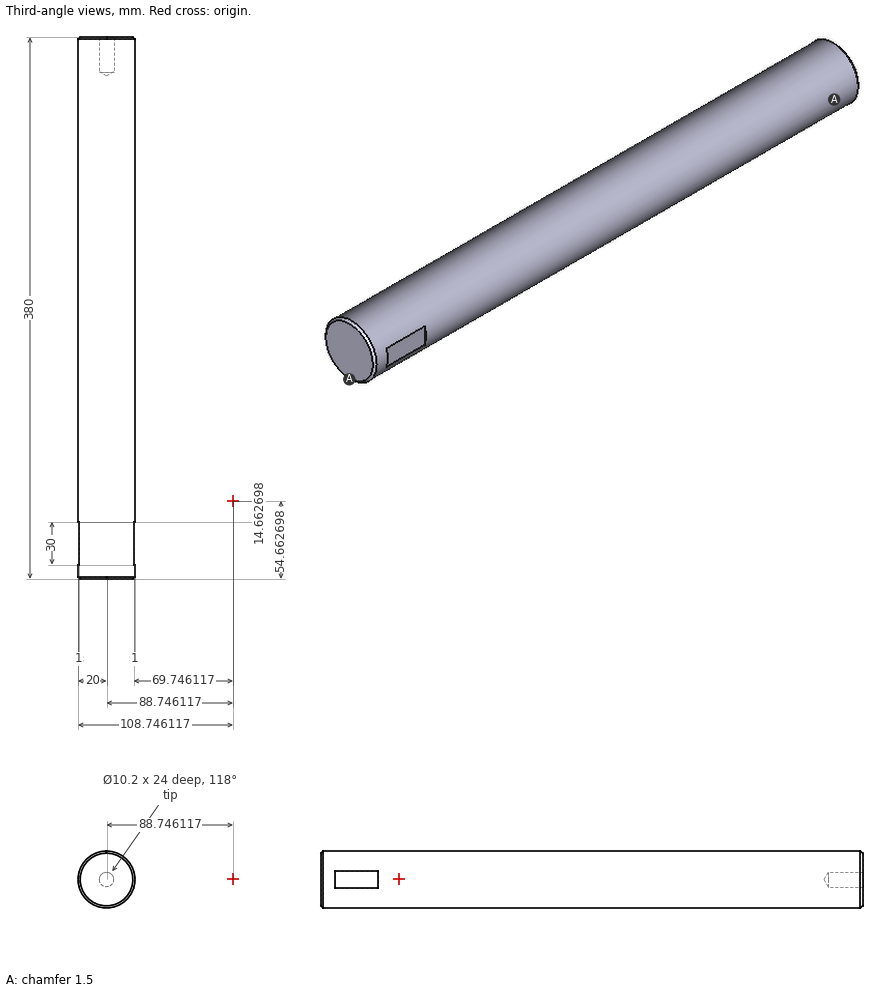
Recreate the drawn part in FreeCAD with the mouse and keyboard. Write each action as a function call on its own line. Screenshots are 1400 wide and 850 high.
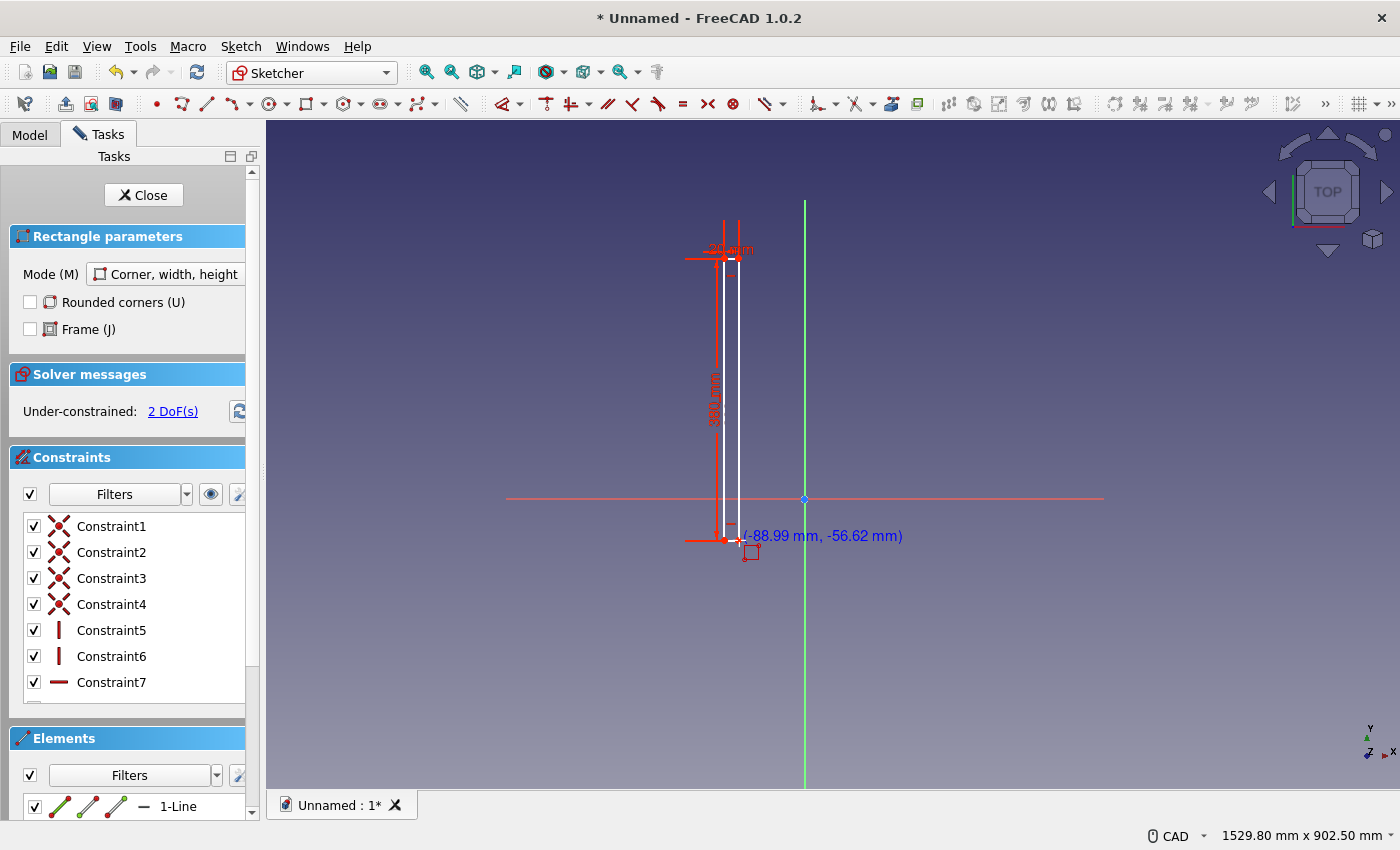
key(g)
key(l)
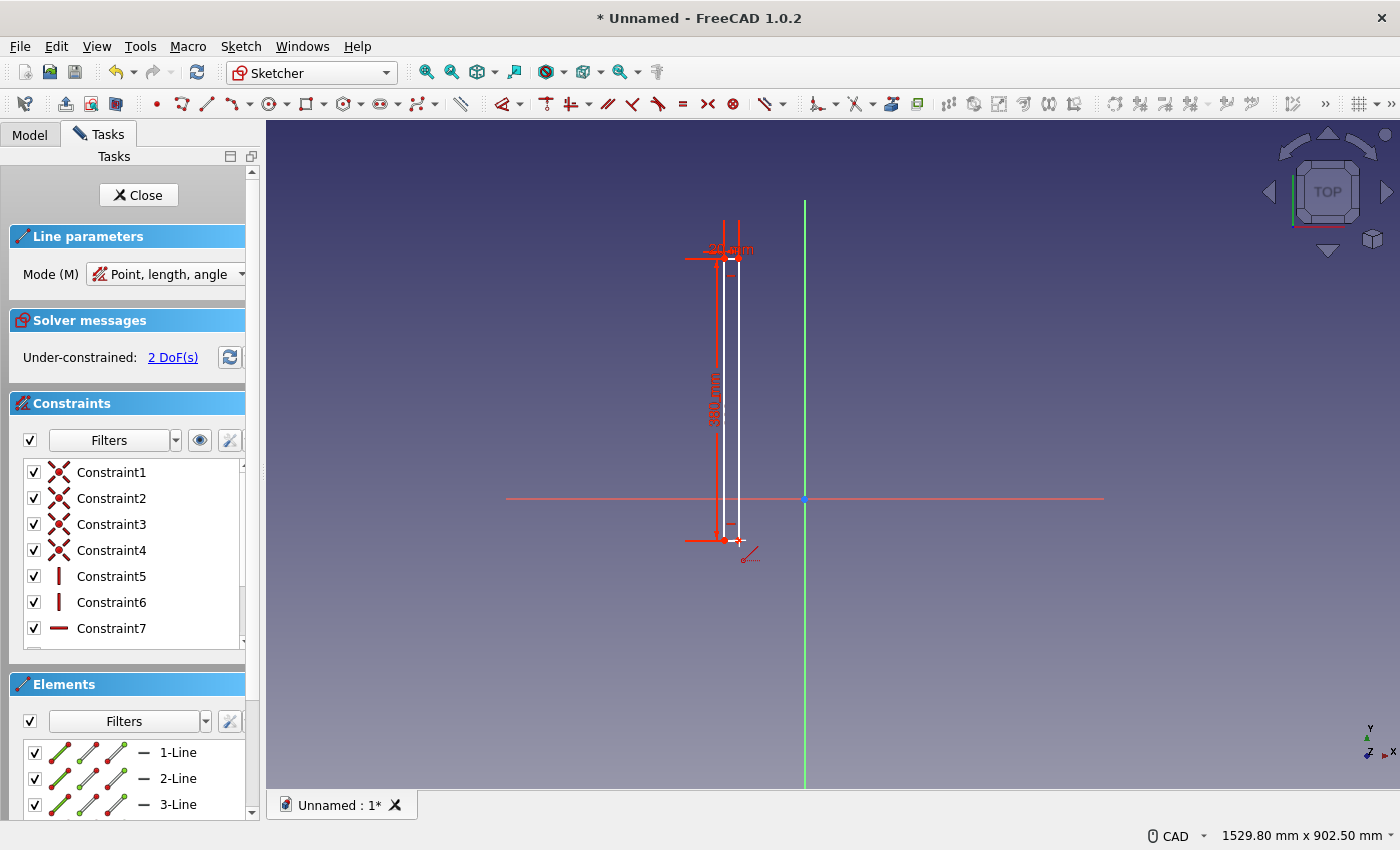
click(739, 568)
click(739, 652)
key(Escape)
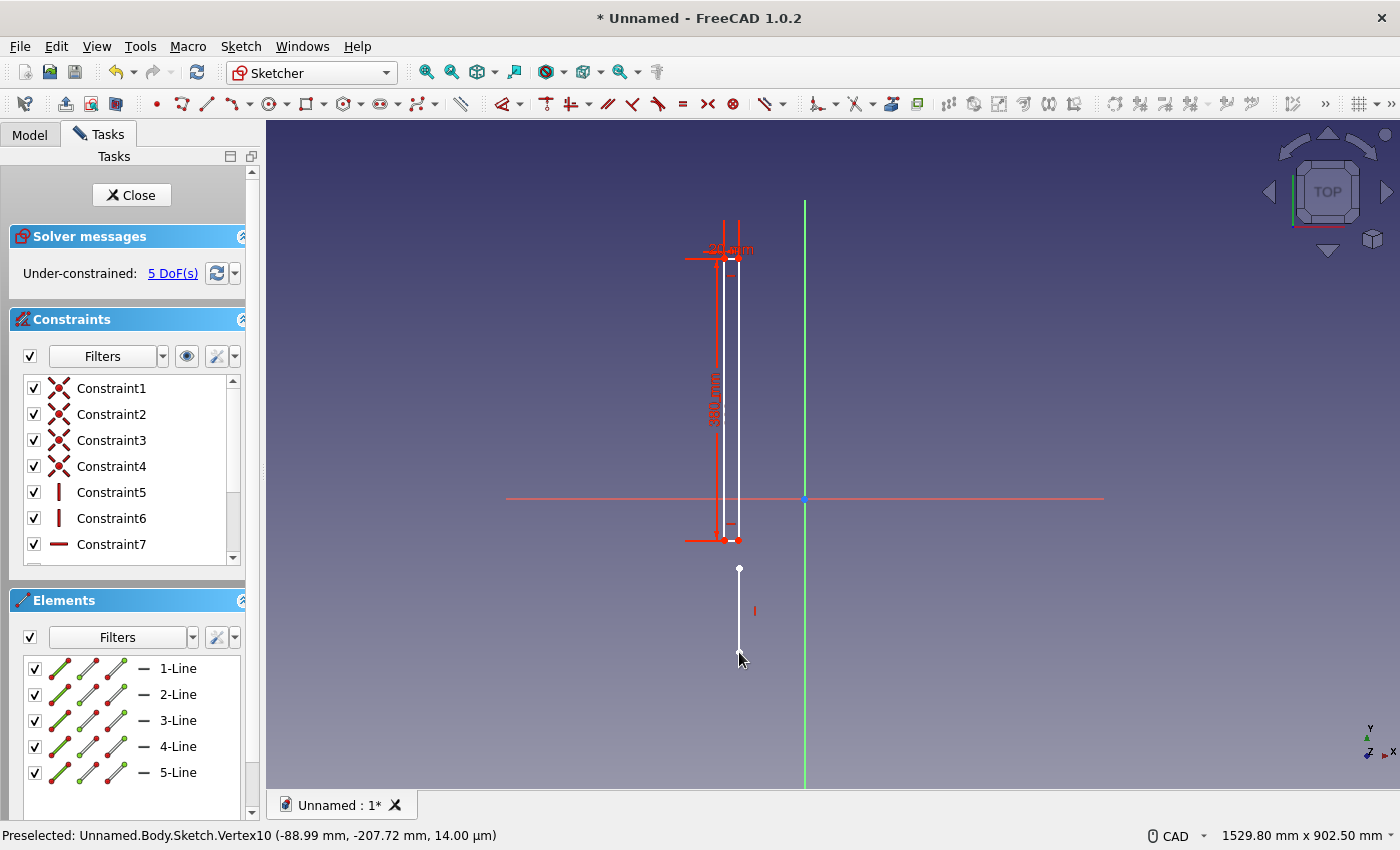
click(739, 594)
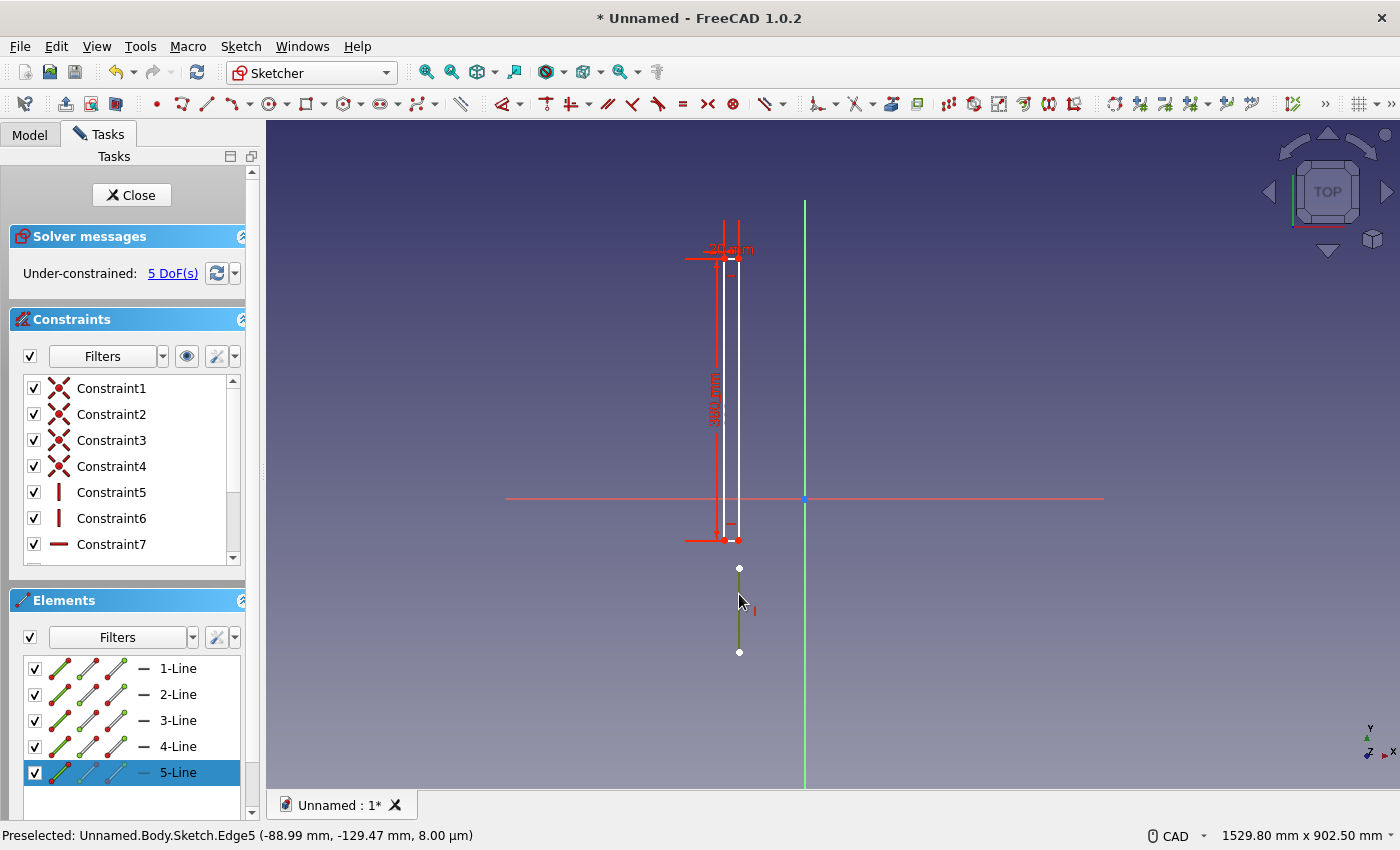
click(461, 104)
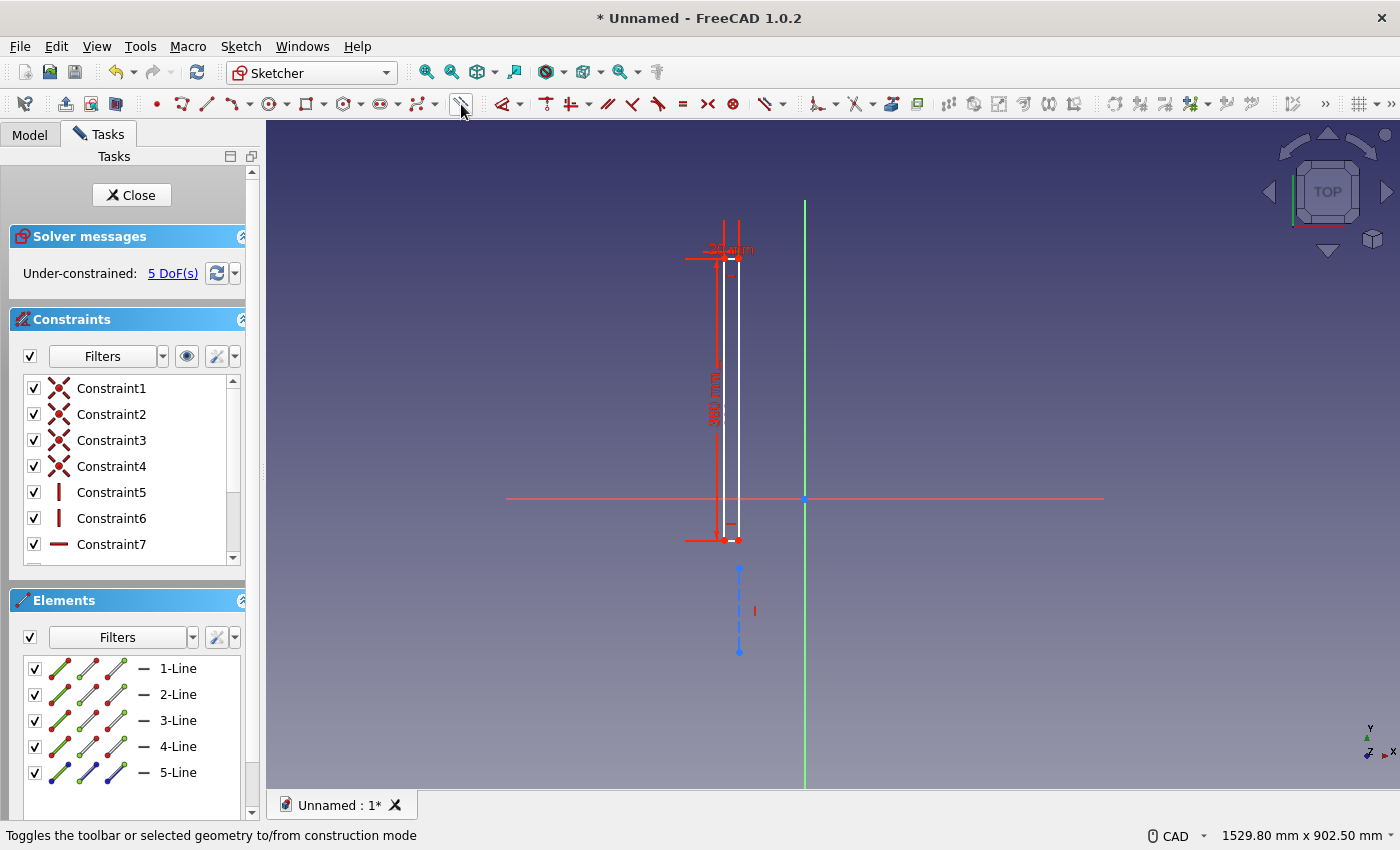
click(502, 104)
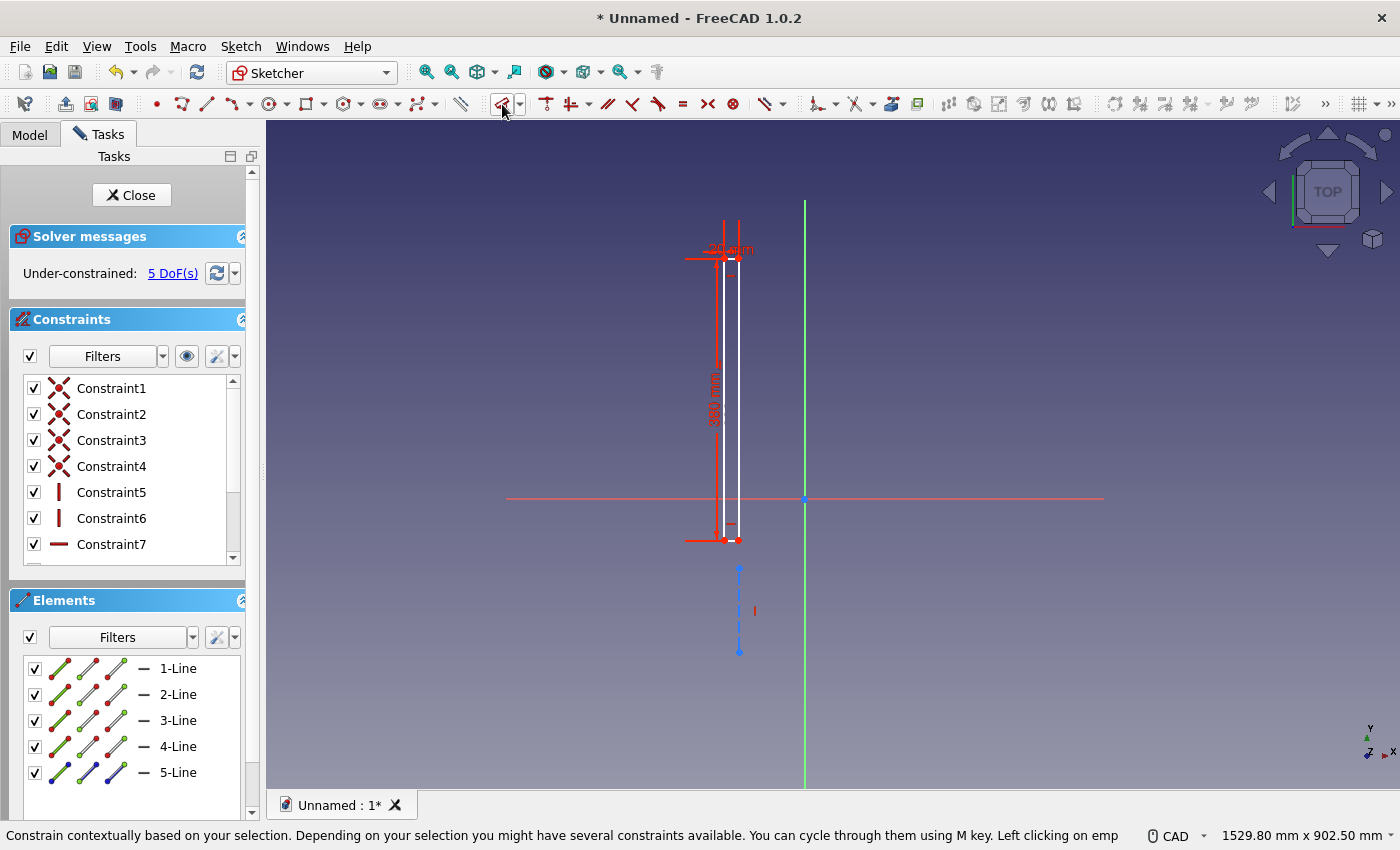
click(724, 541)
click(690, 520)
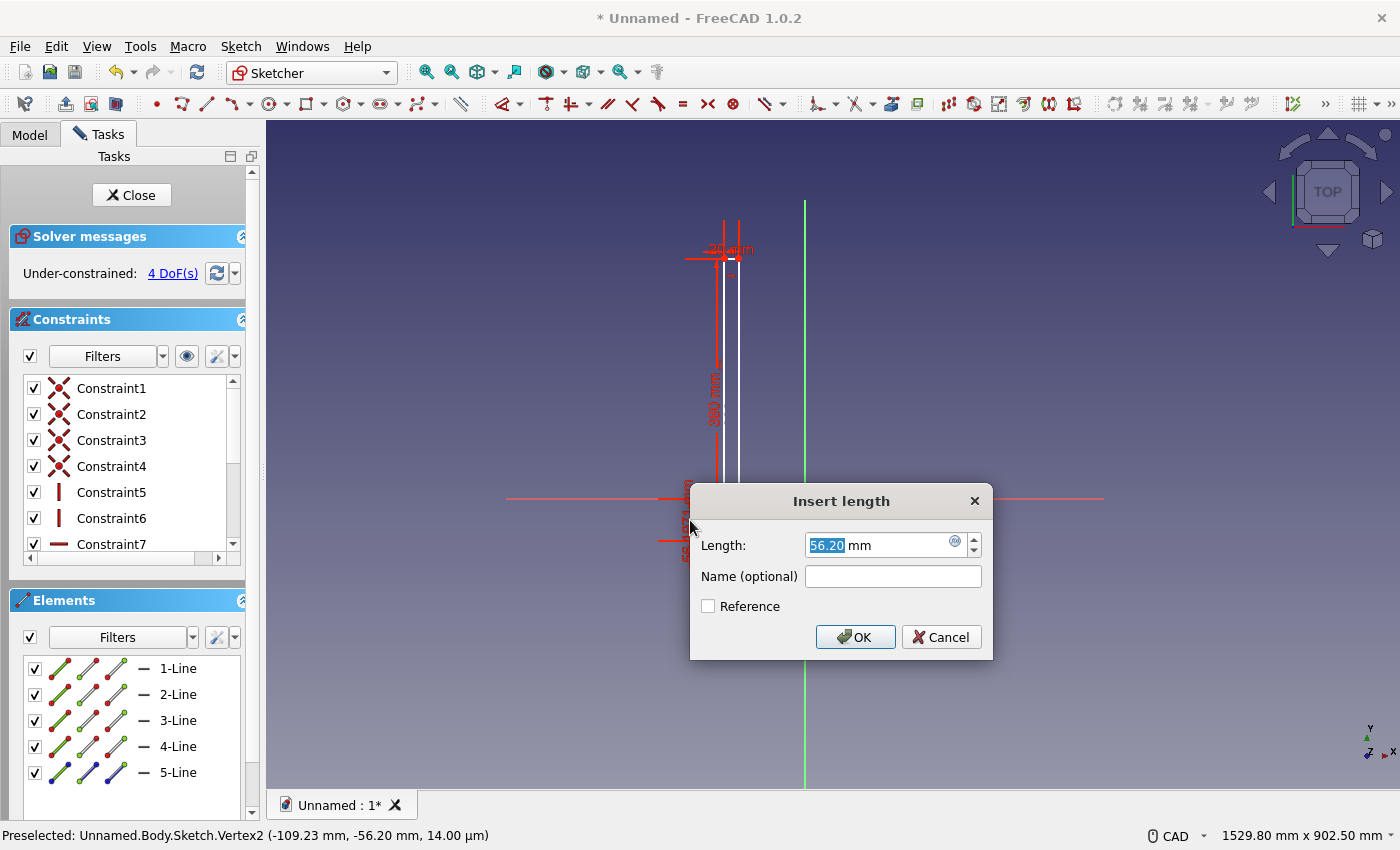
text(54.662698)
key(Return)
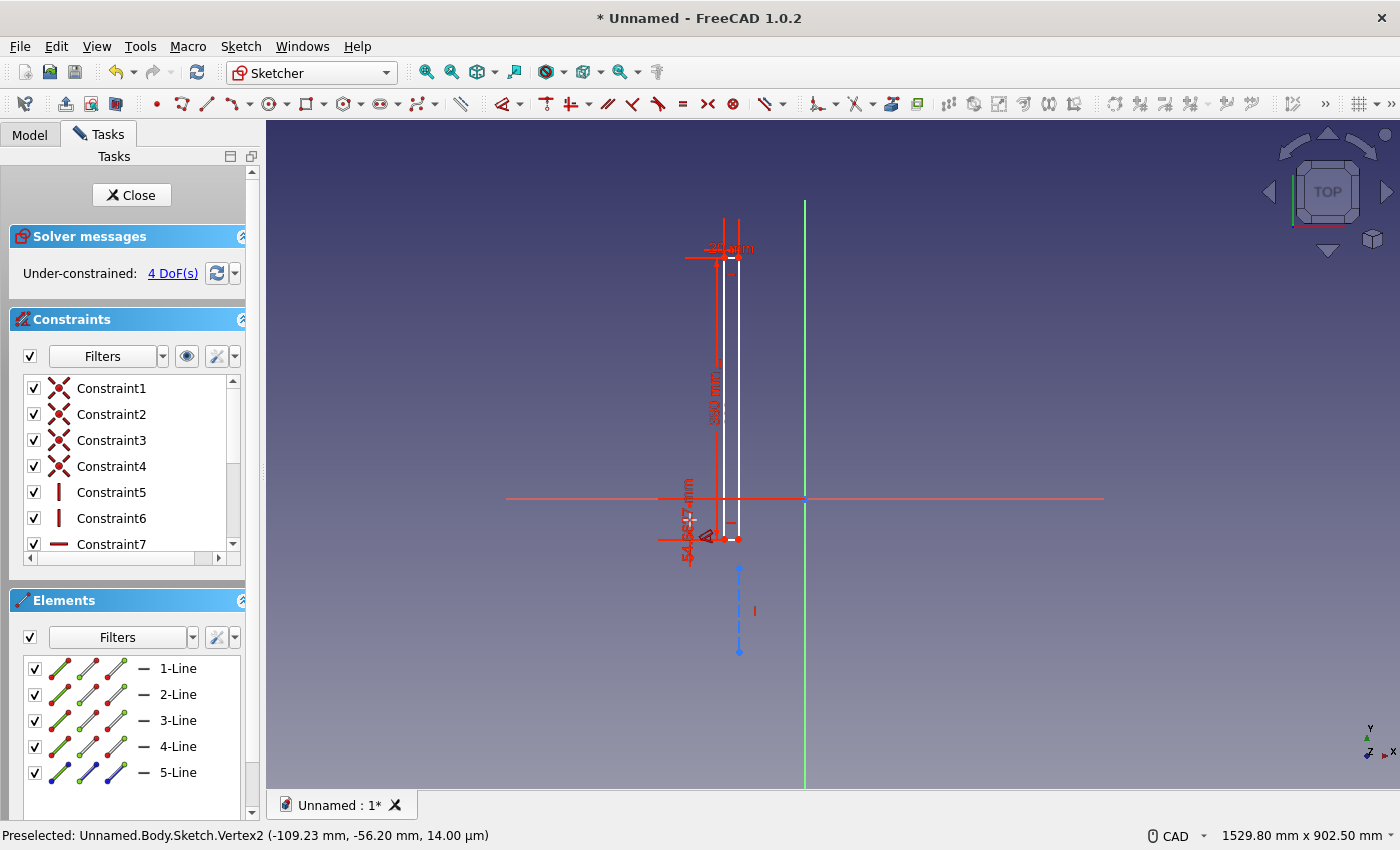
click(739, 540)
click(772, 574)